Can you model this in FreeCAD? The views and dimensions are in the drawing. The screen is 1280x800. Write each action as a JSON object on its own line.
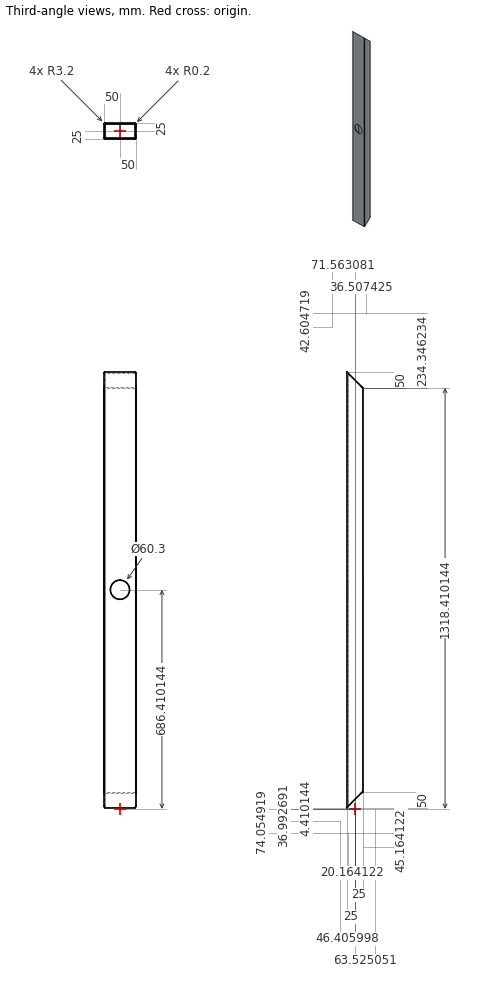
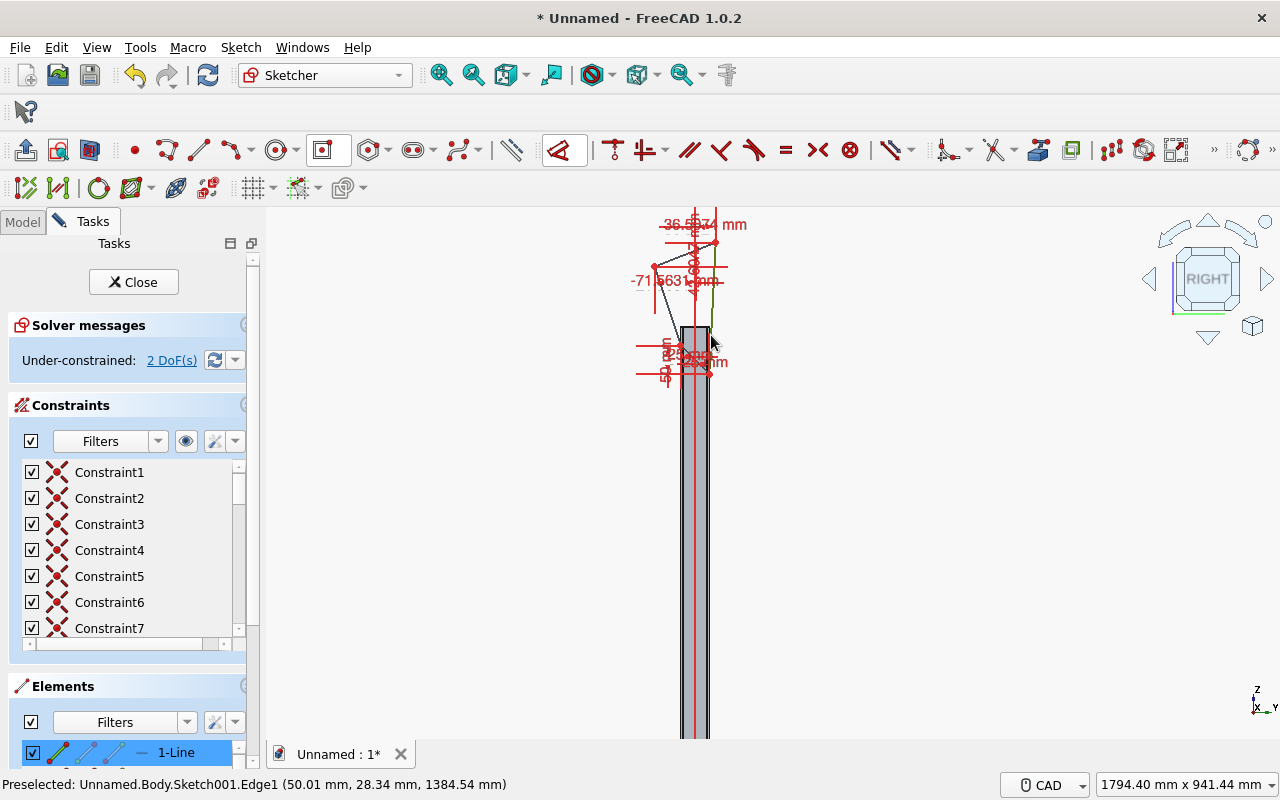
{"action": "left_click", "coordinate": [582, 150]}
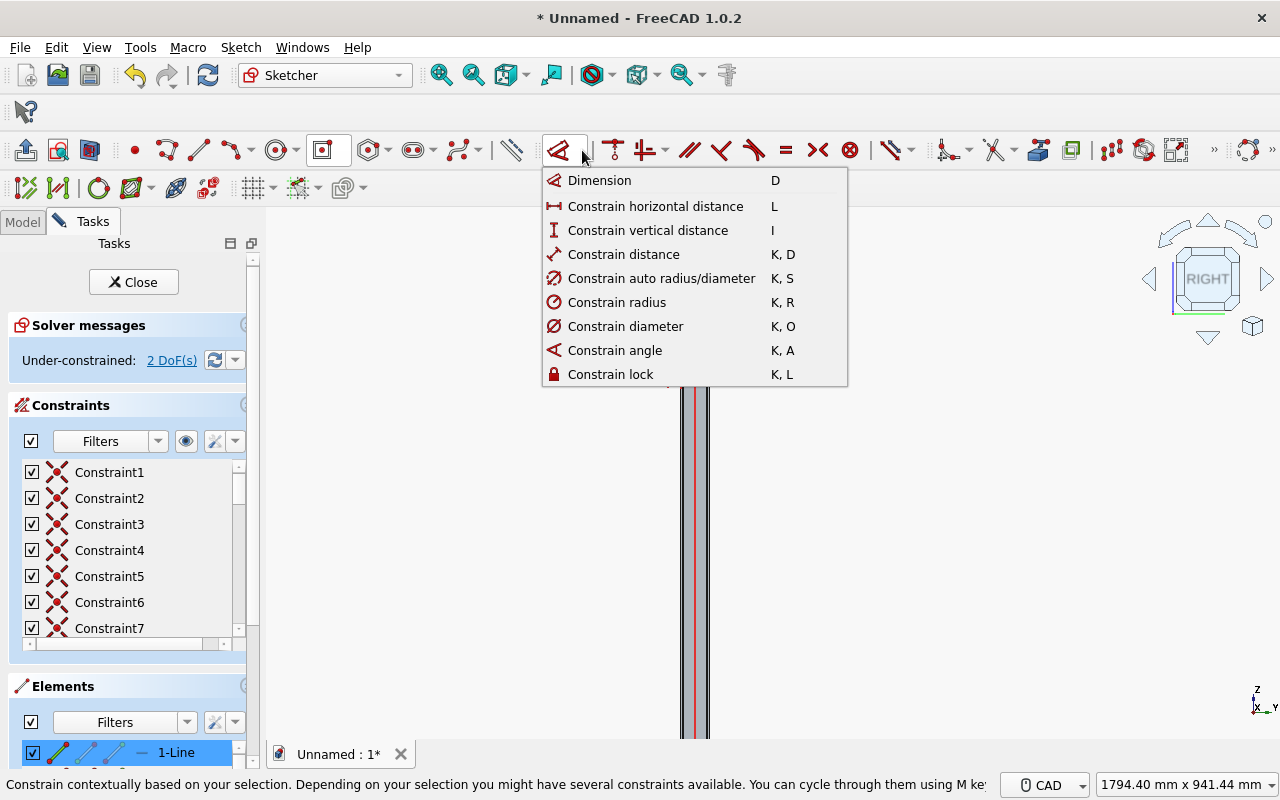
{"action": "left_click", "coordinate": [695, 230]}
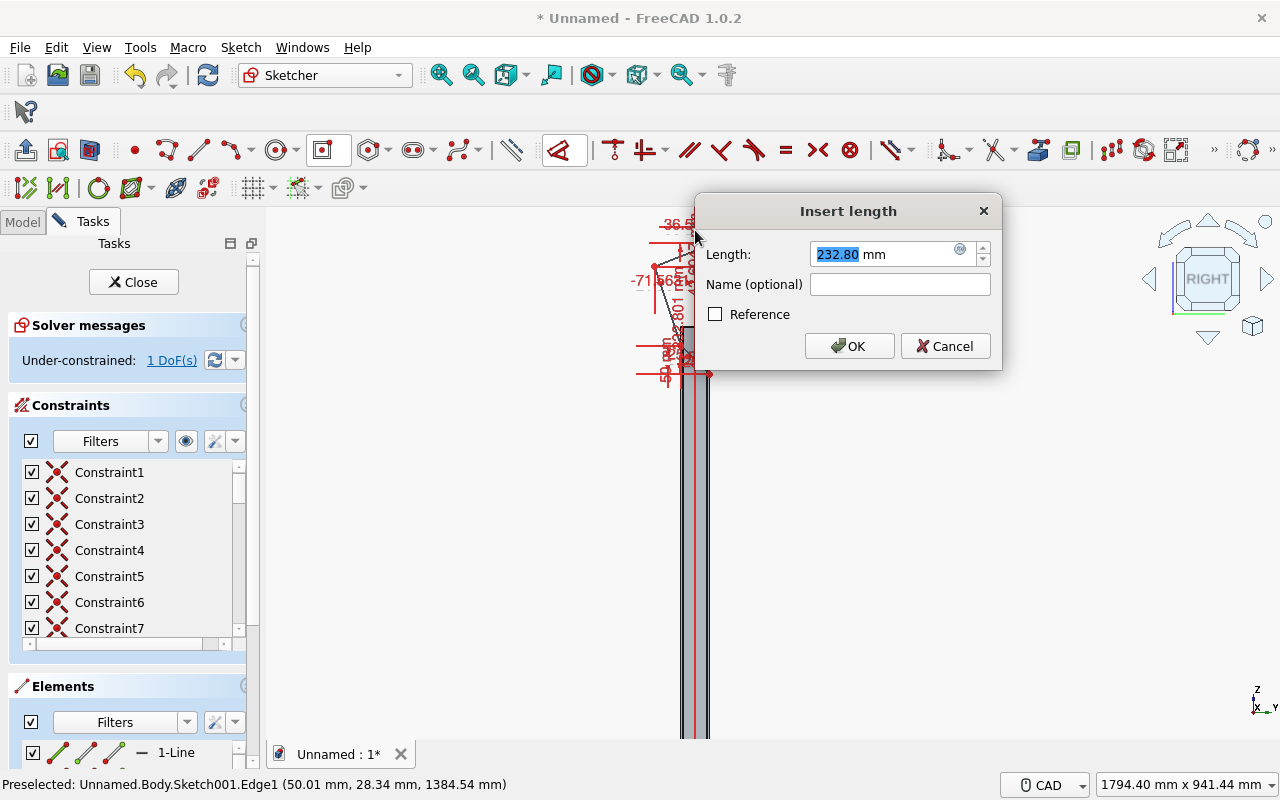
{"action": "type", "text": "234.346234"}
{"action": "key", "text": "Return"}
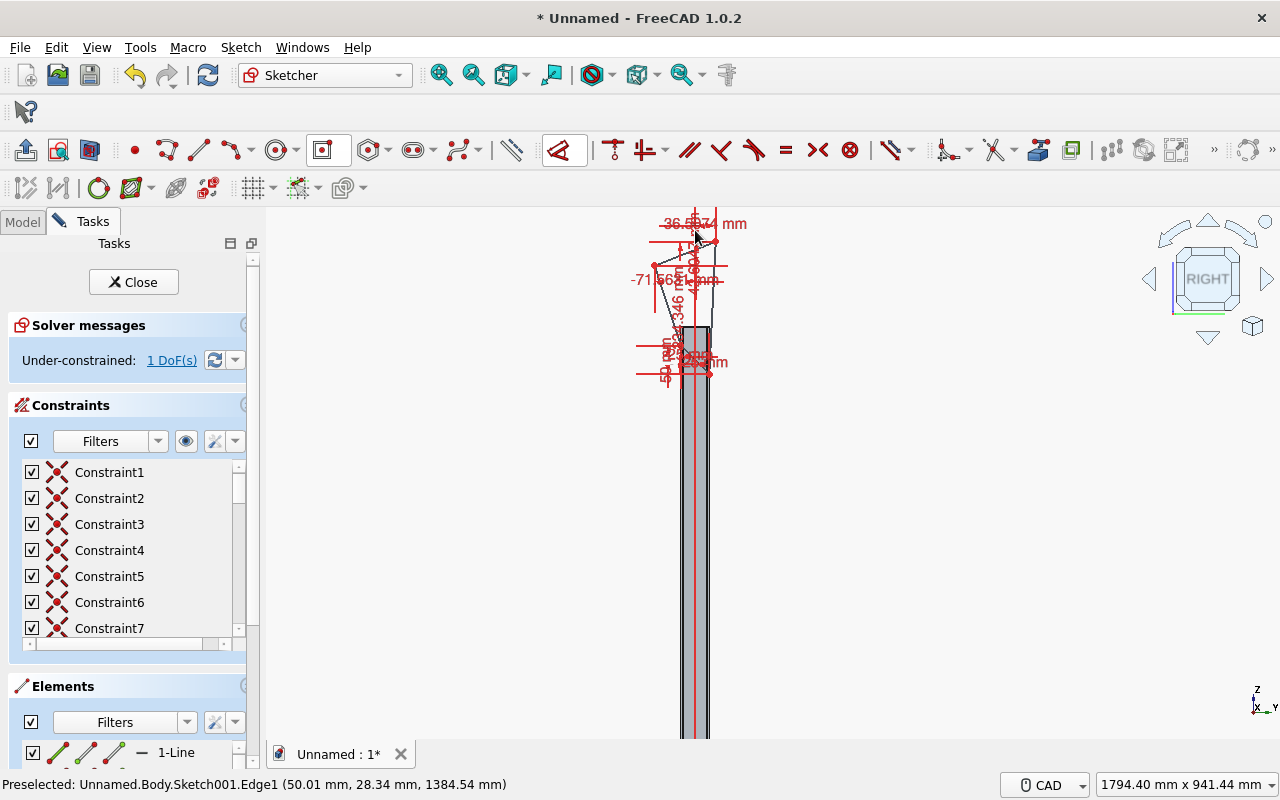
{"action": "left_click", "coordinate": [709, 374]}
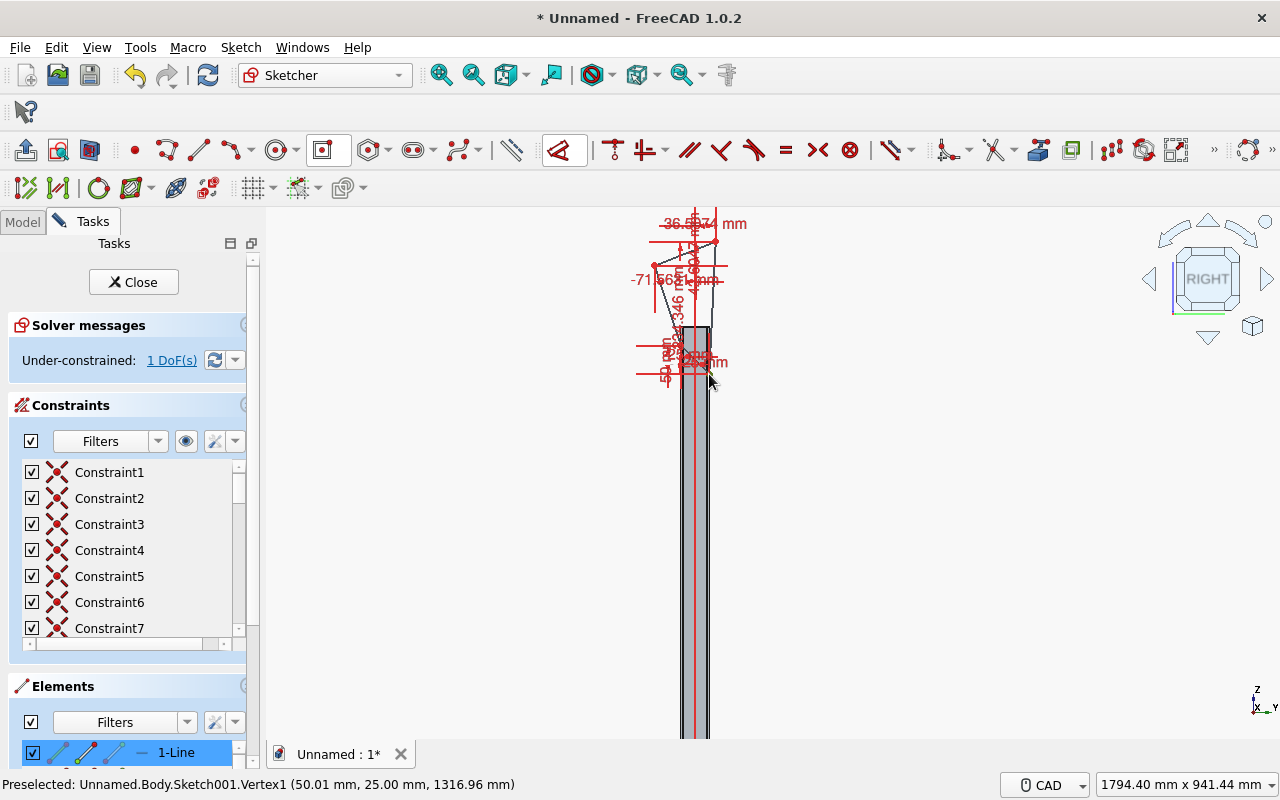
{"action": "left_click", "coordinate": [582, 150]}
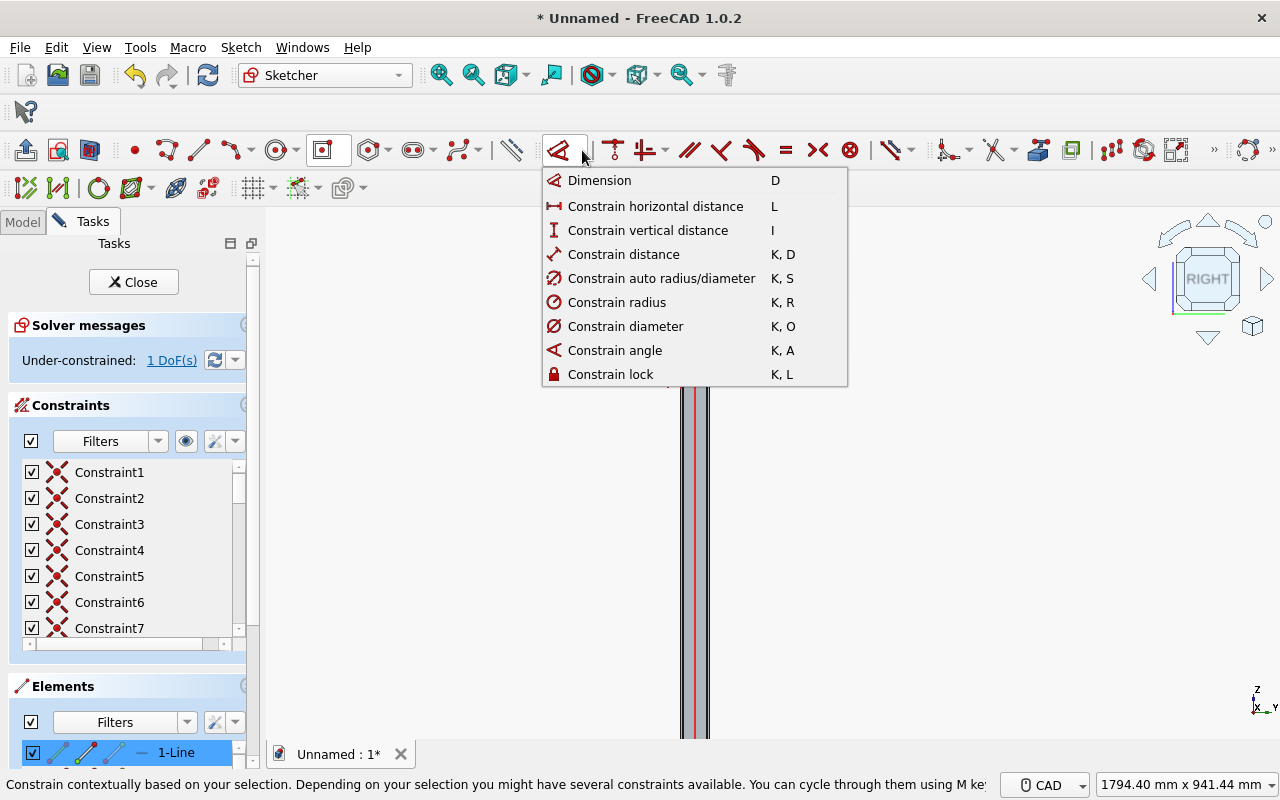
{"action": "left_click", "coordinate": [695, 230]}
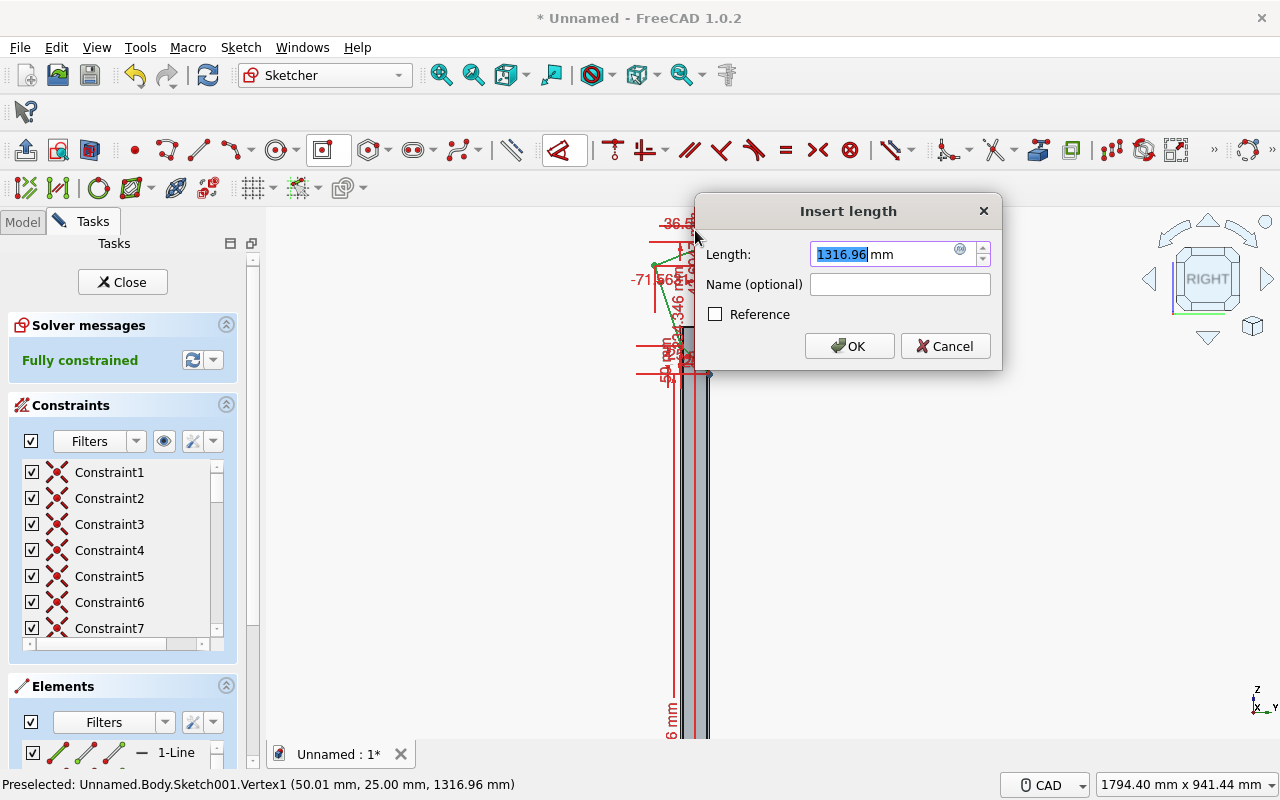
{"action": "type", "text": "1318.410144"}
{"action": "key", "text": "Return"}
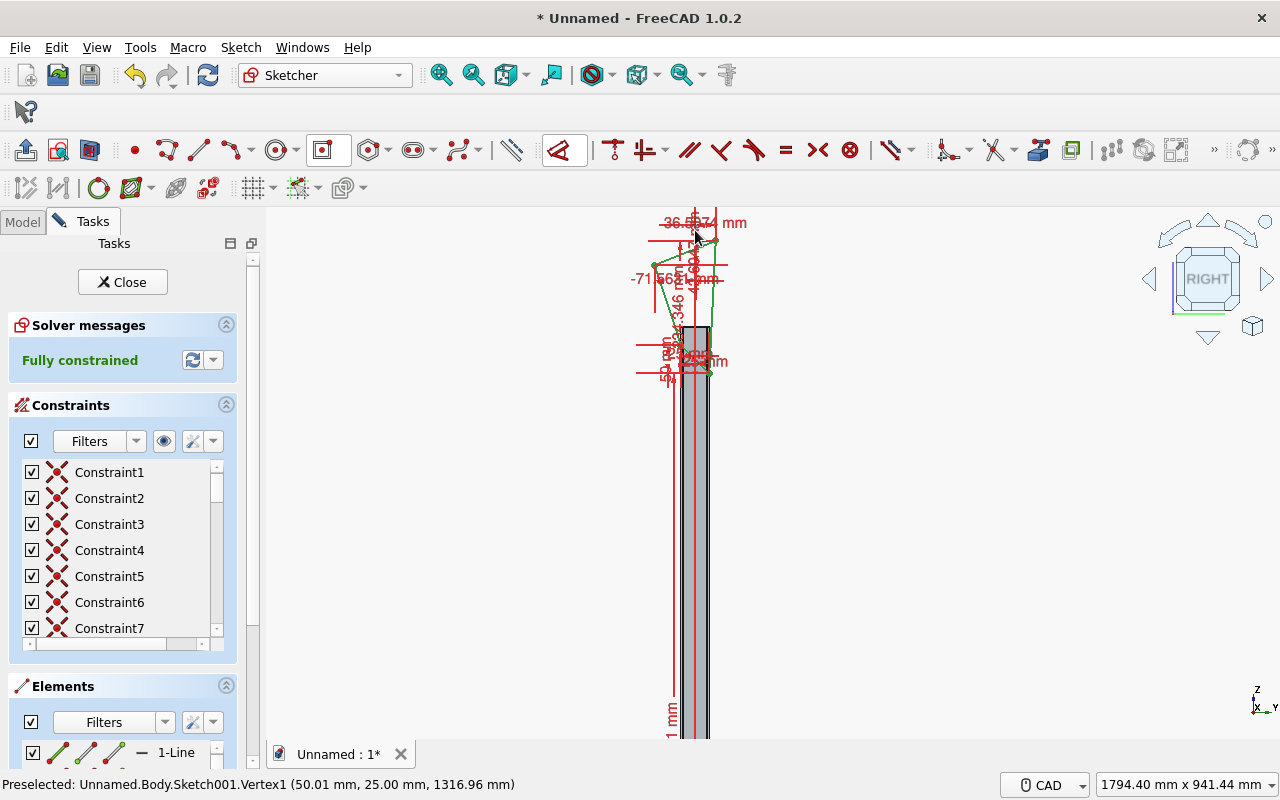
{"action": "left_click", "coordinate": [123, 282]}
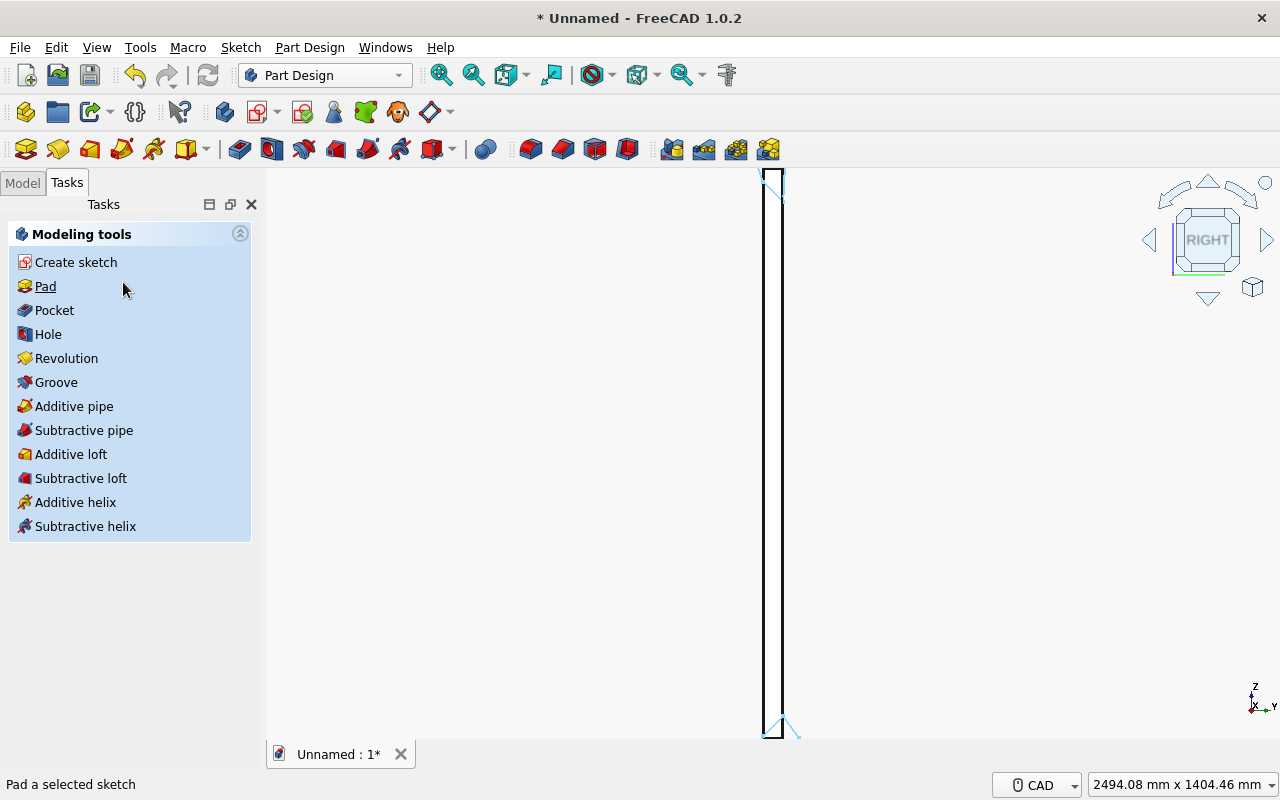
{"action": "left_click", "coordinate": [240, 150]}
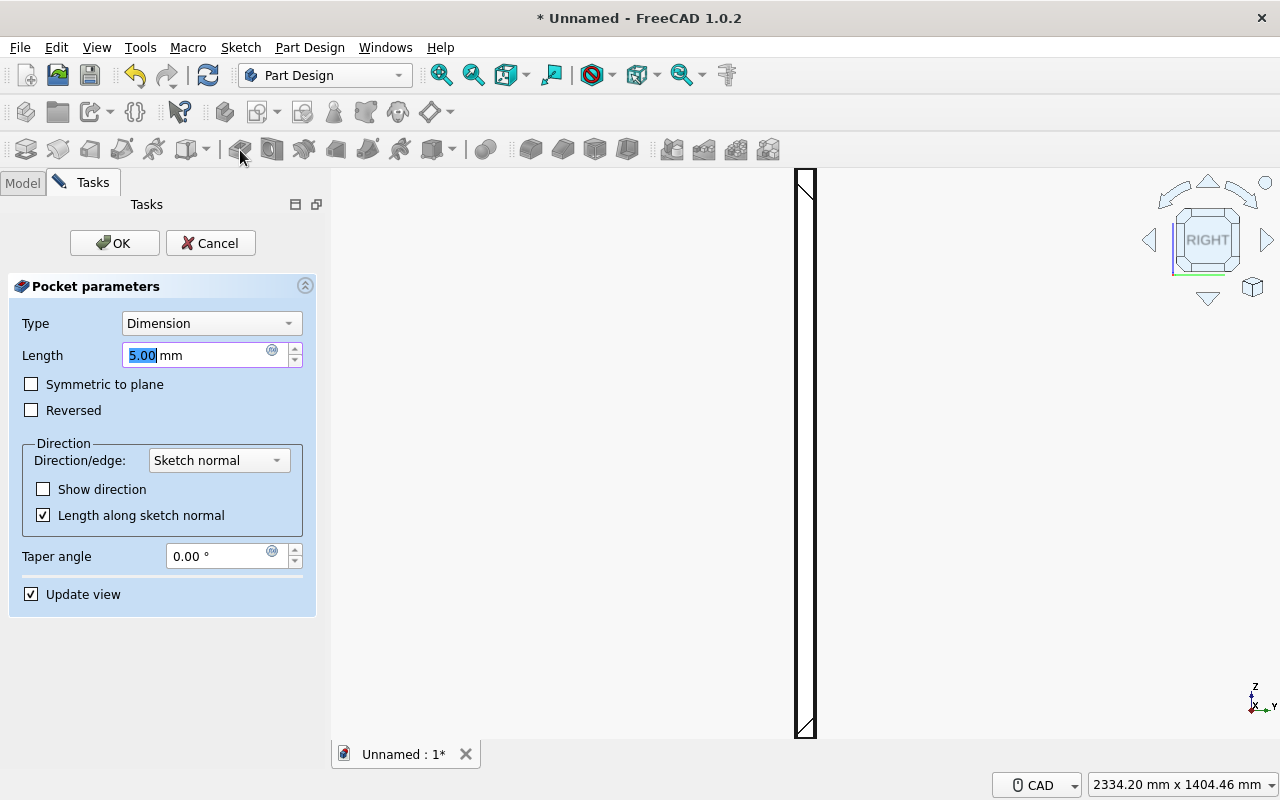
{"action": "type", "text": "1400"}
{"action": "key", "text": "Tab"}